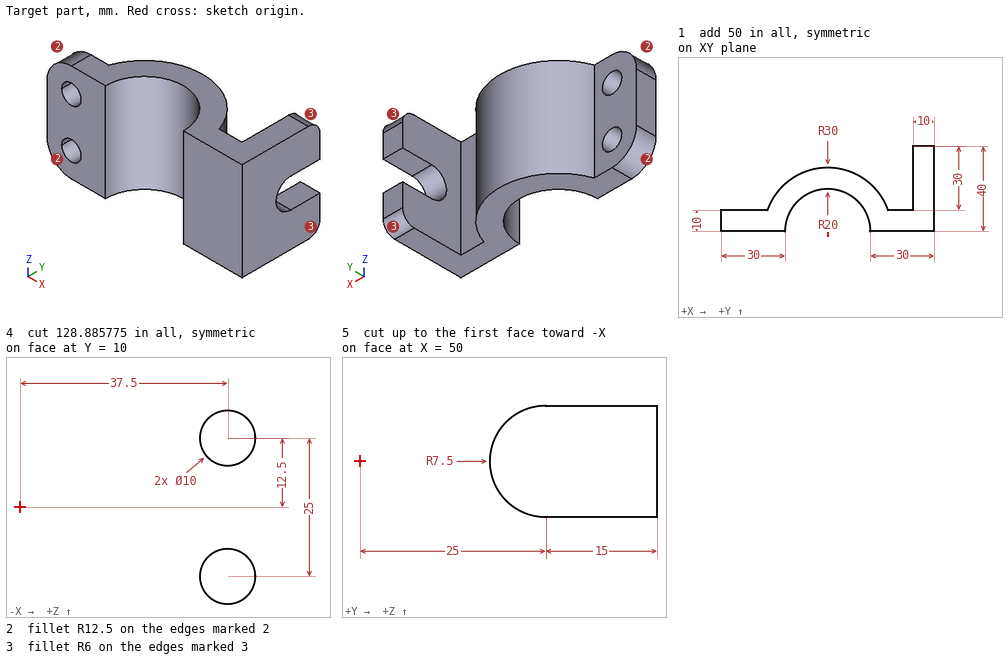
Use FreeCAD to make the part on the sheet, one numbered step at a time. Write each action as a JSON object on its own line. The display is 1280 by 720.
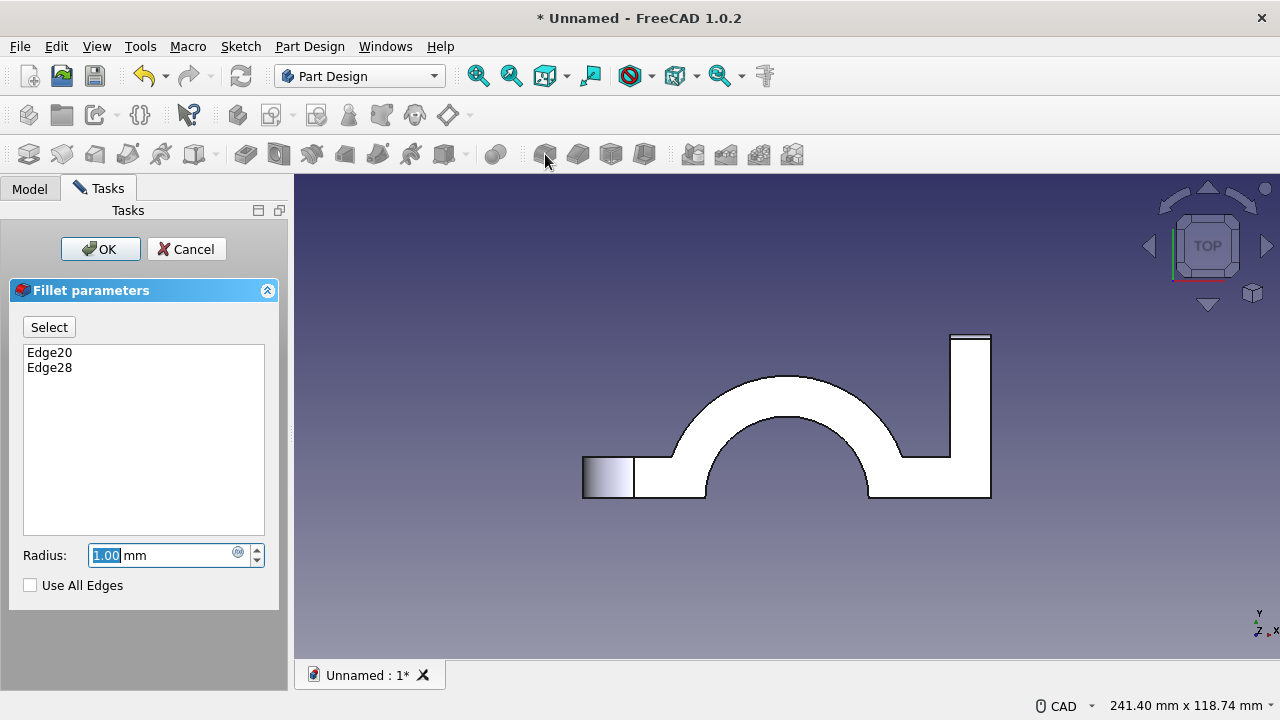
{"action": "type", "text": "6"}
{"action": "key", "text": "Tab"}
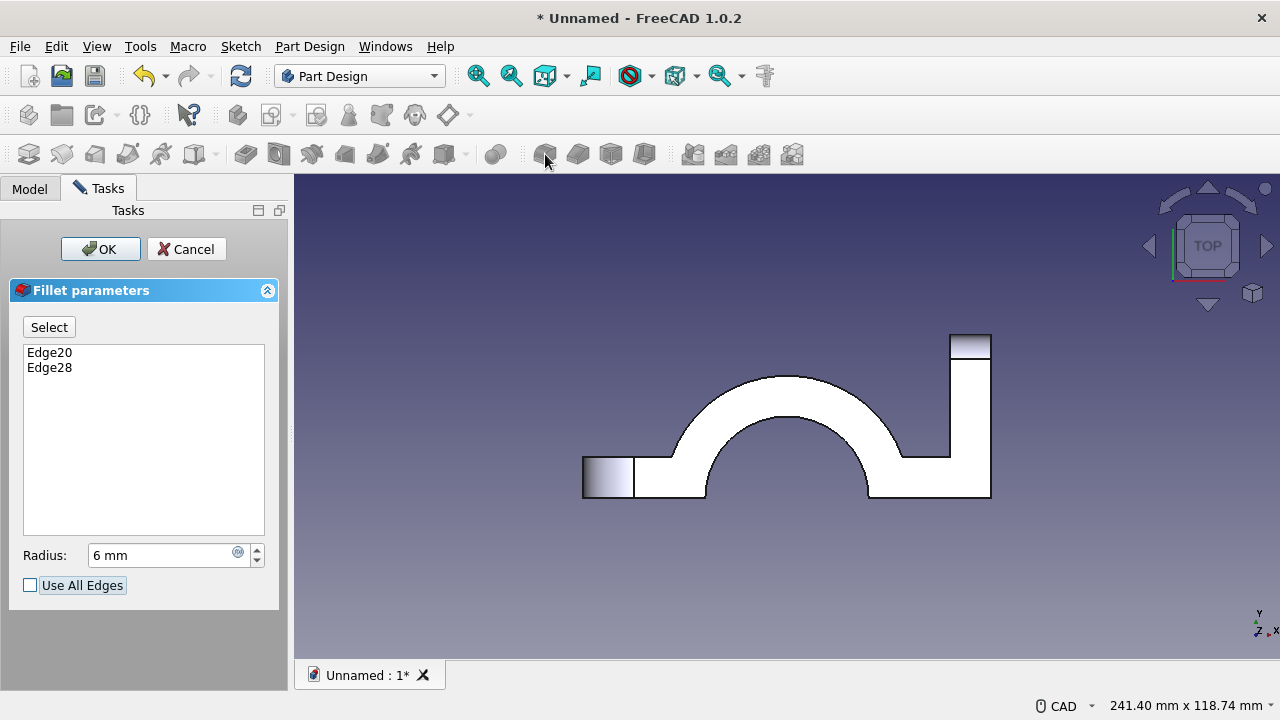
{"action": "left_click", "coordinate": [101, 249]}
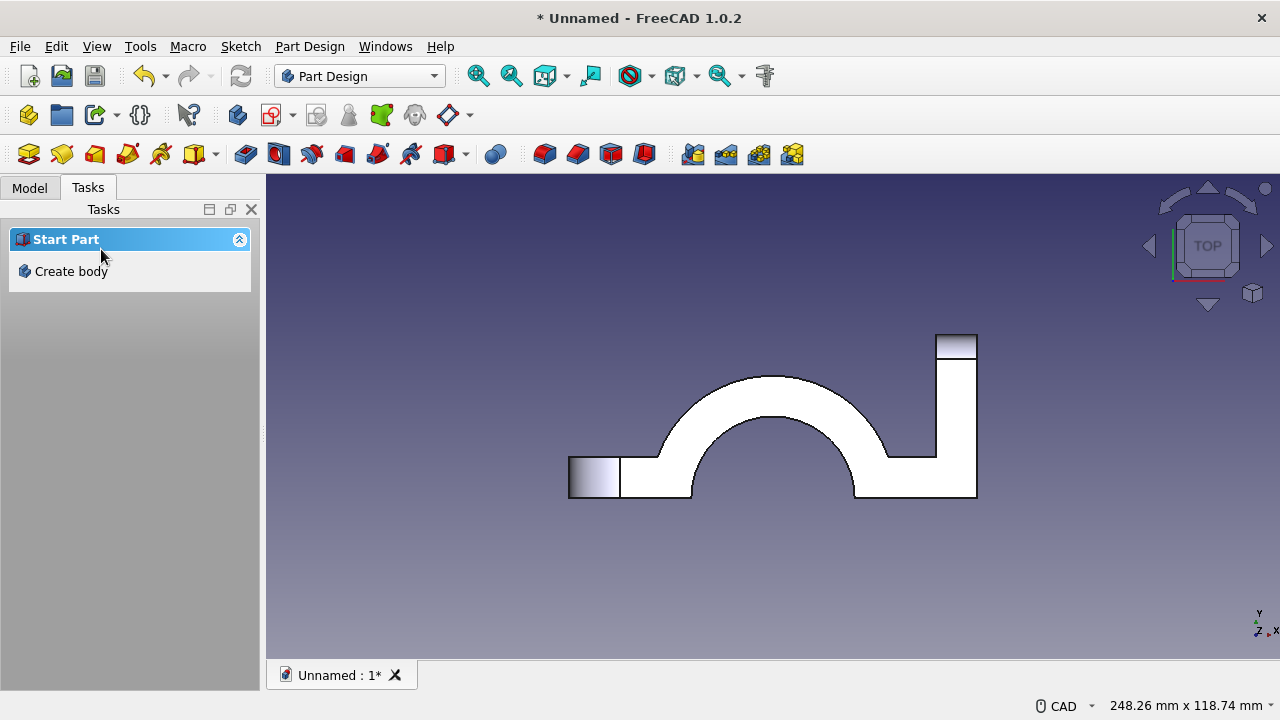
{"action": "left_click", "coordinate": [479, 76]}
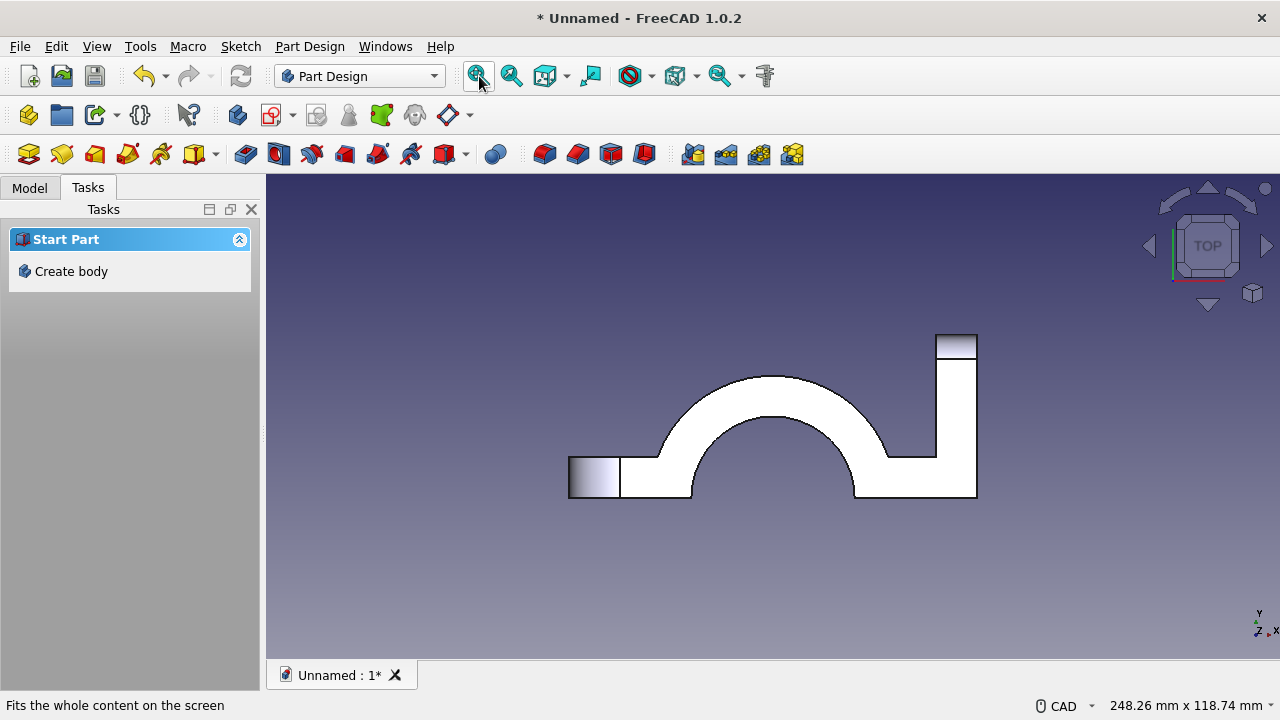
{"action": "key", "text": "4"}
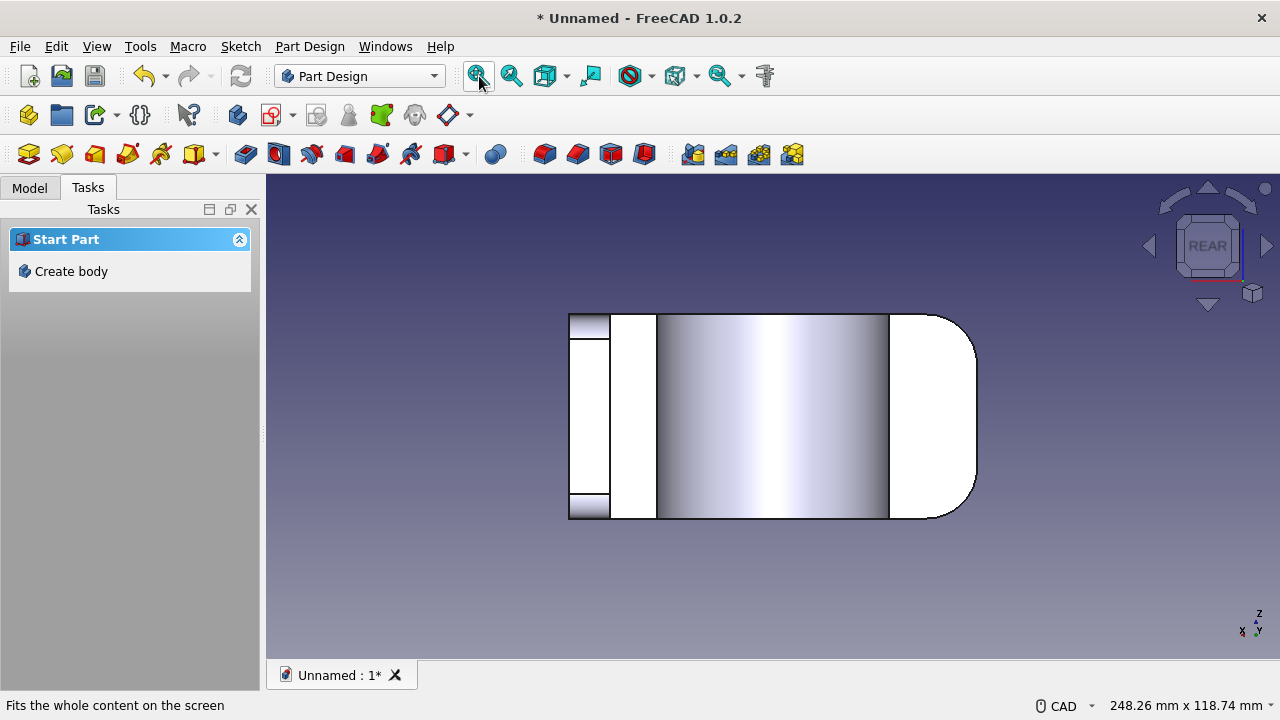
{"action": "left_click", "coordinate": [479, 76]}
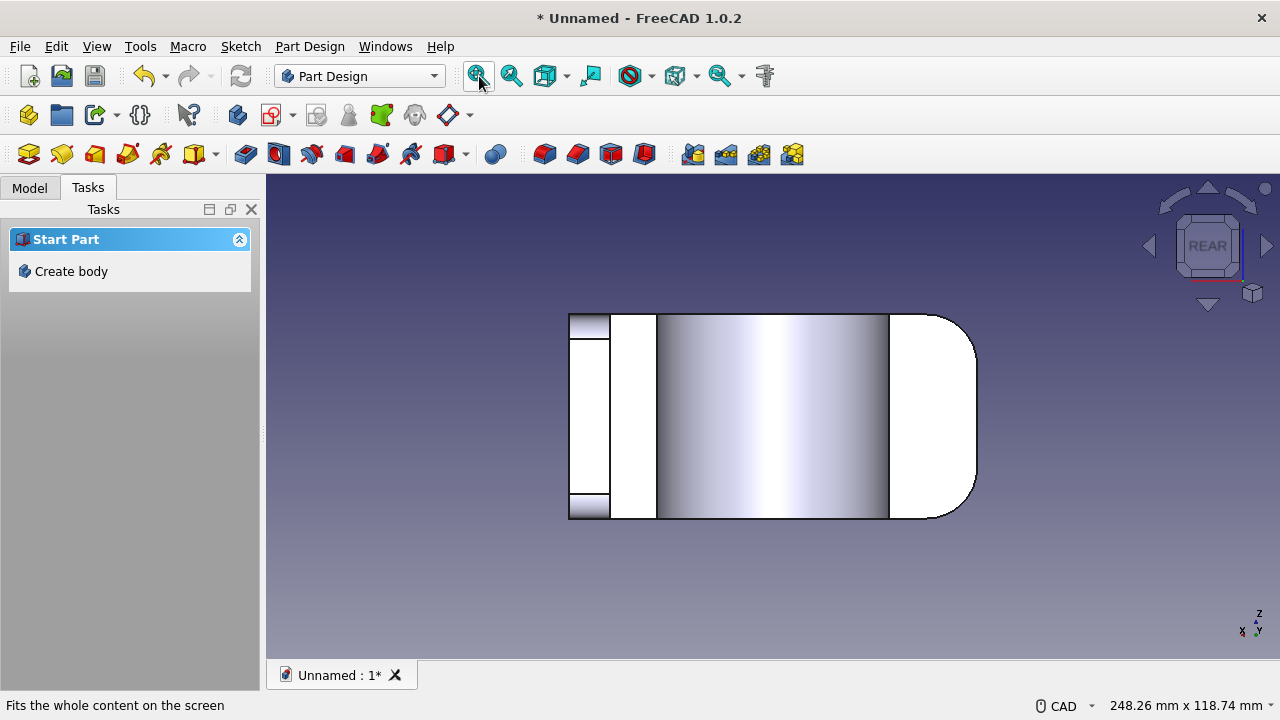
{"action": "left_click", "coordinate": [933, 386]}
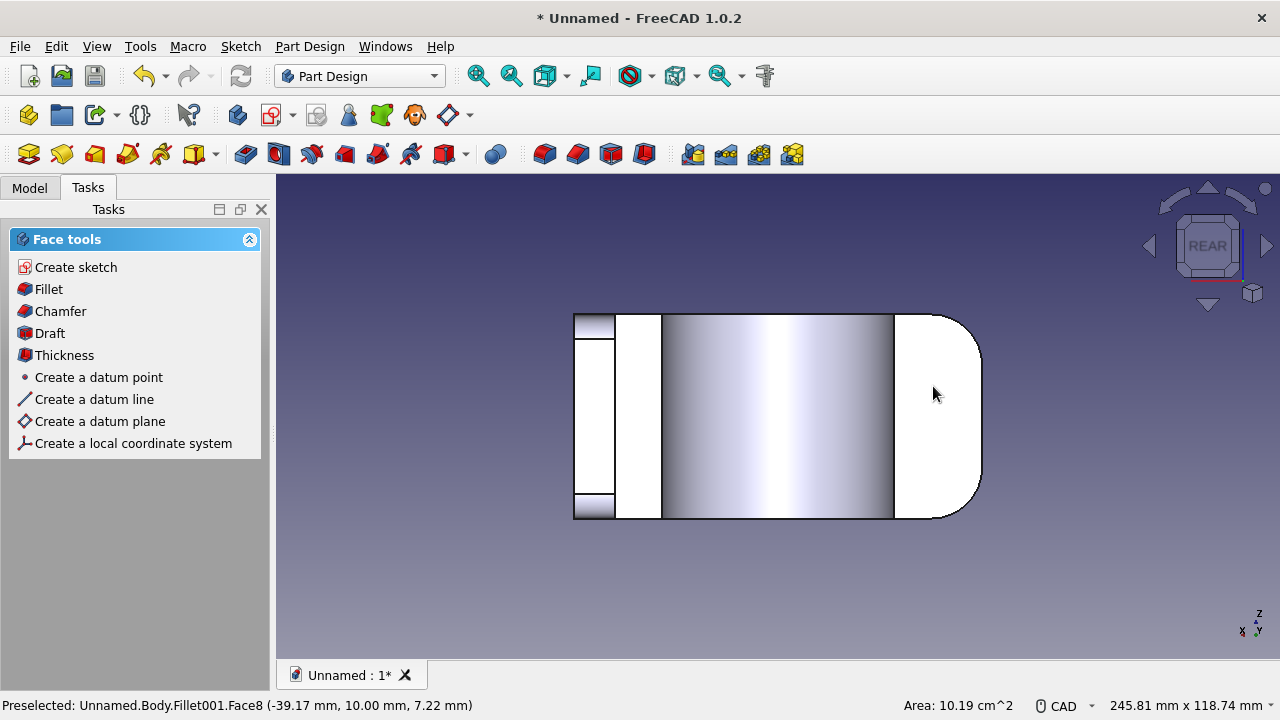
{"action": "left_click", "coordinate": [270, 116]}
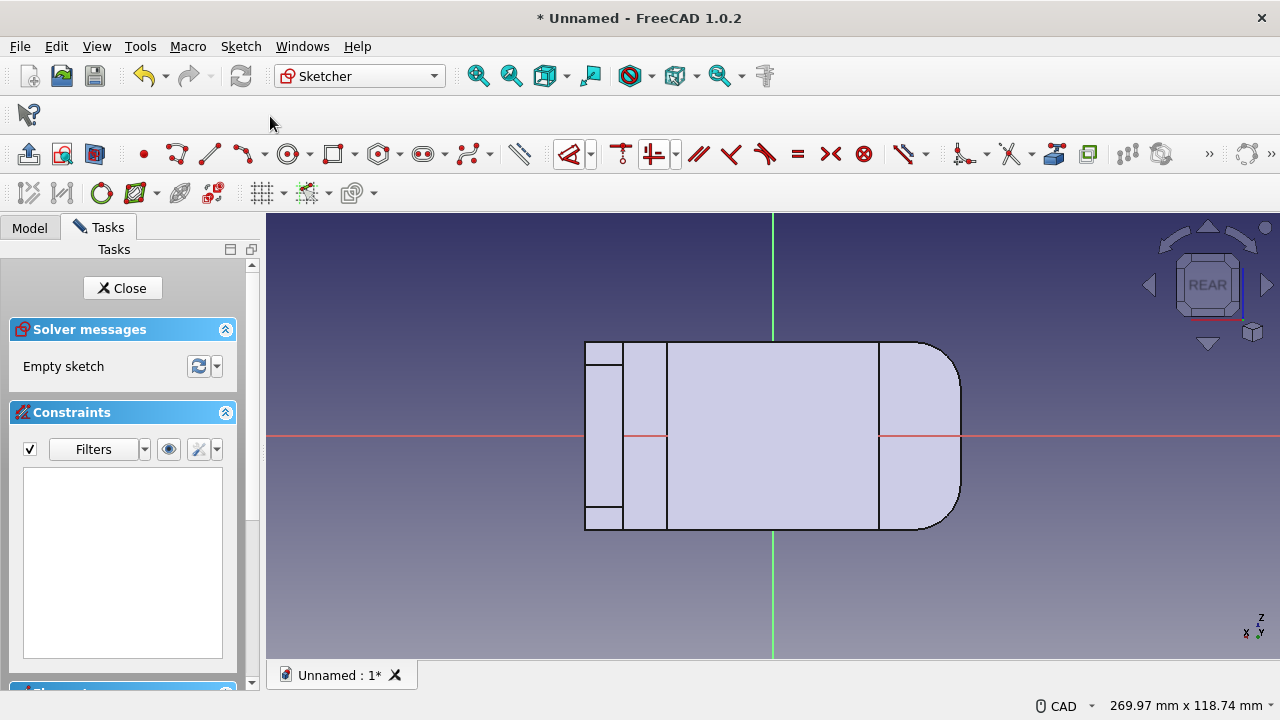
{"action": "left_click", "coordinate": [95, 154]}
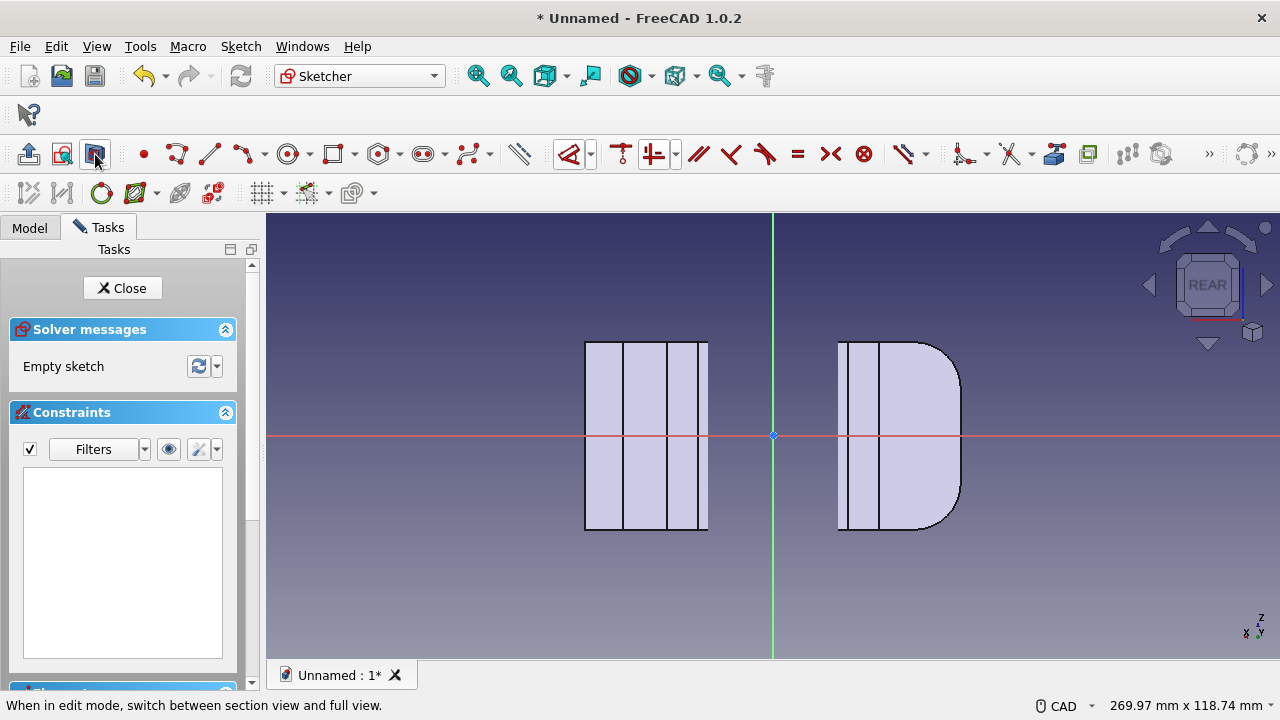
{"action": "scroll", "coordinate": [974, 436], "scroll_direction": "up", "scroll_amount": 4}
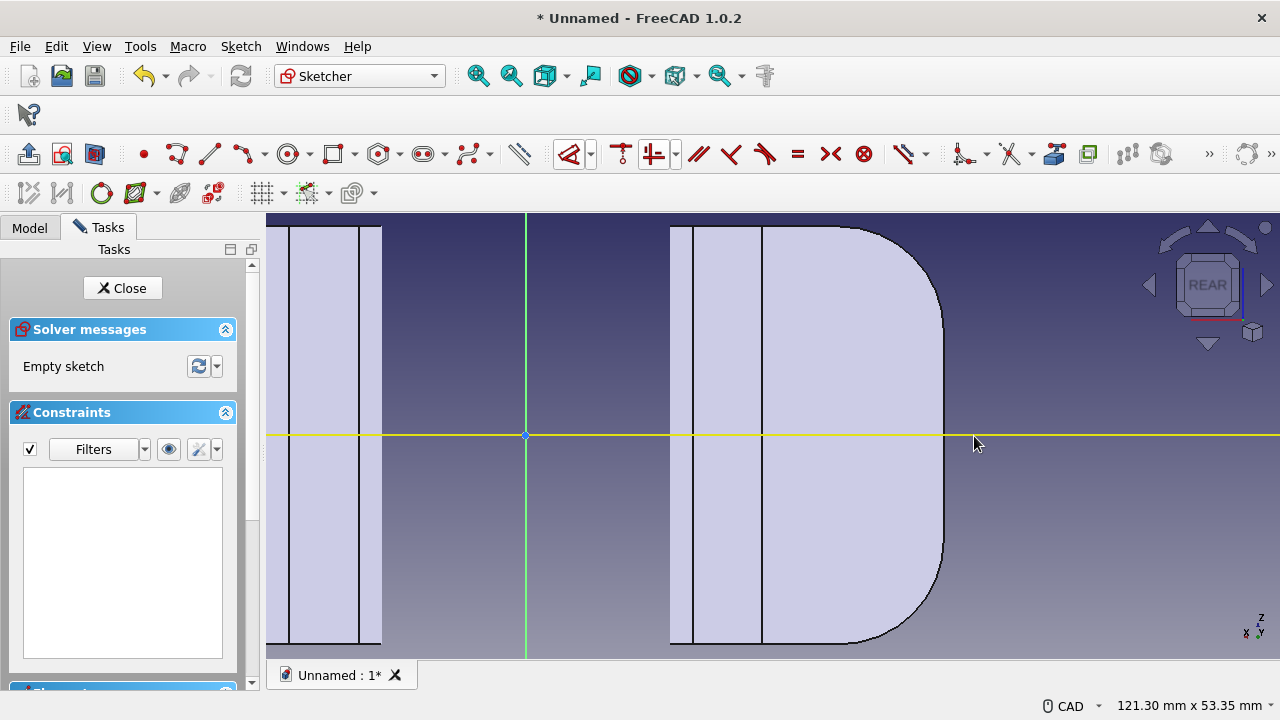
{"action": "left_click", "coordinate": [288, 154]}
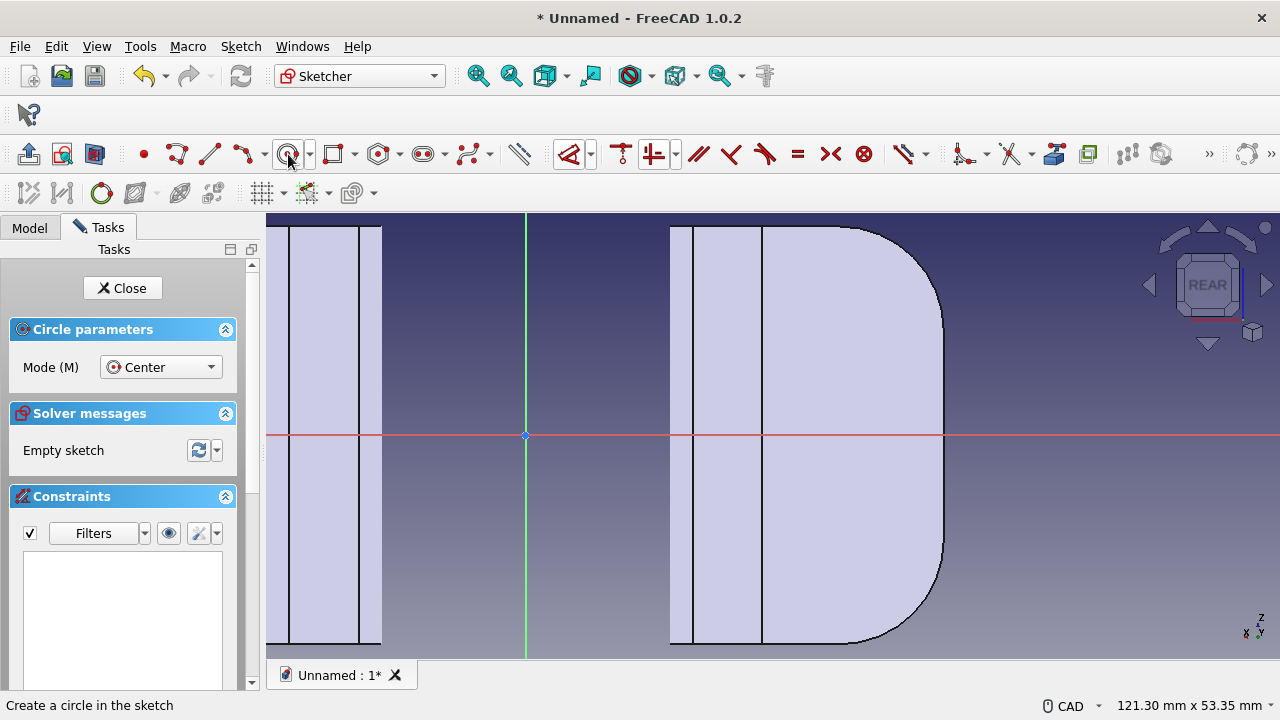
{"action": "left_click", "coordinate": [839, 331]}
{"action": "left_click", "coordinate": [869, 301]}